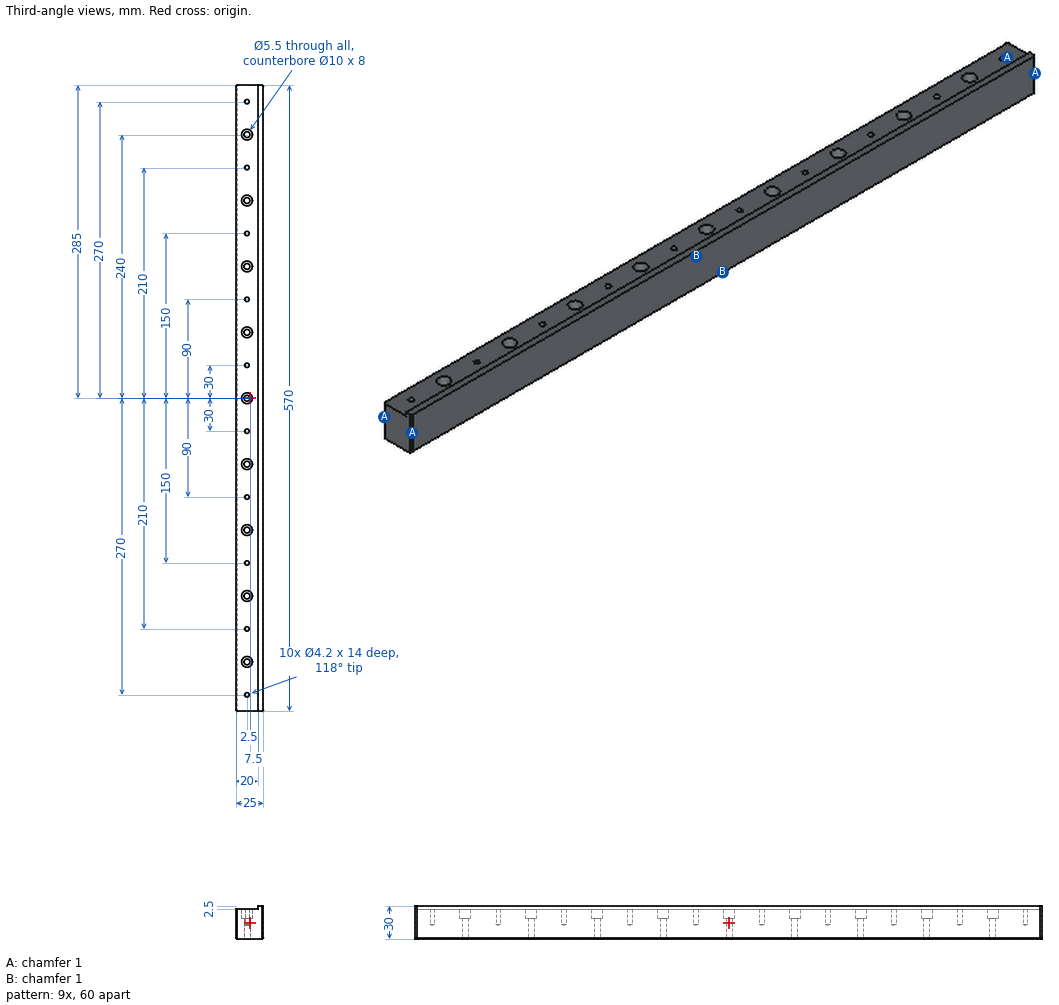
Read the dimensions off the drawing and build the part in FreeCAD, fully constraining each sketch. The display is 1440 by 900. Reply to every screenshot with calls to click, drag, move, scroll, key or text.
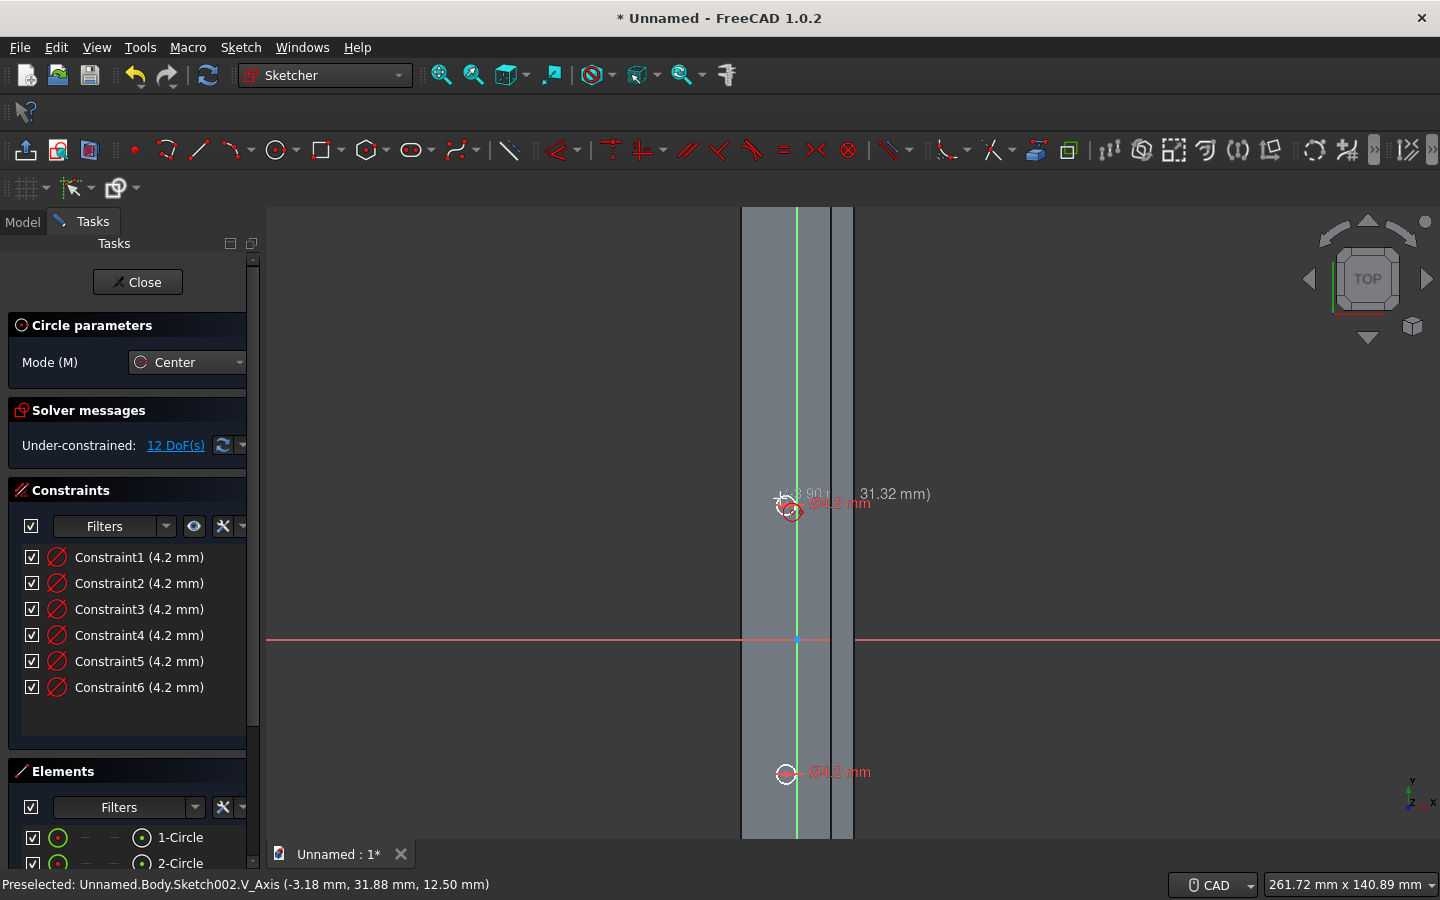
scroll(786, 236, up, 5)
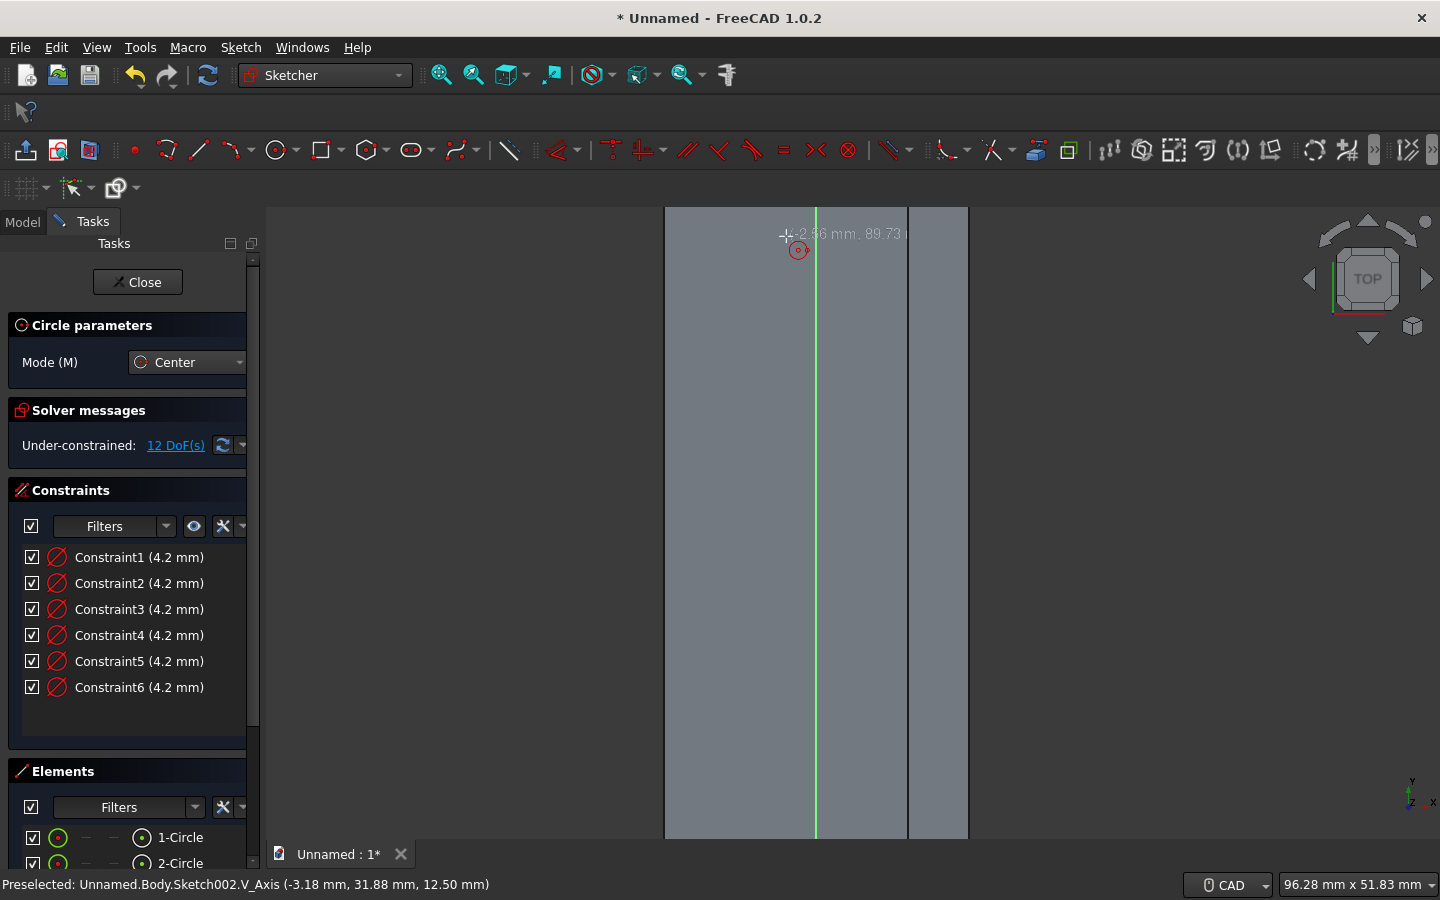
click(786, 235)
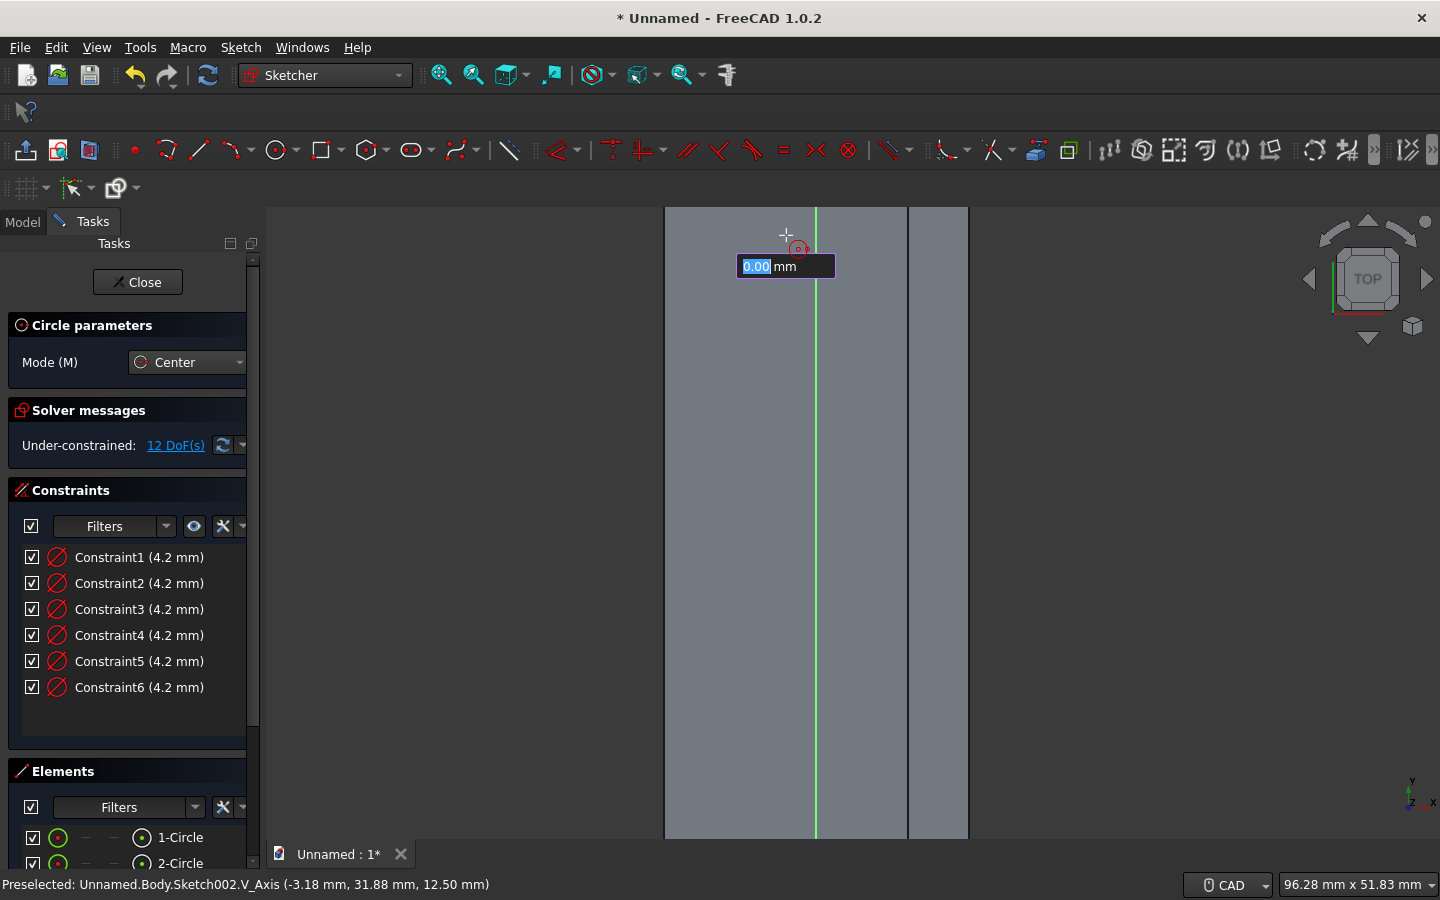
scroll(784, 471, down, 14)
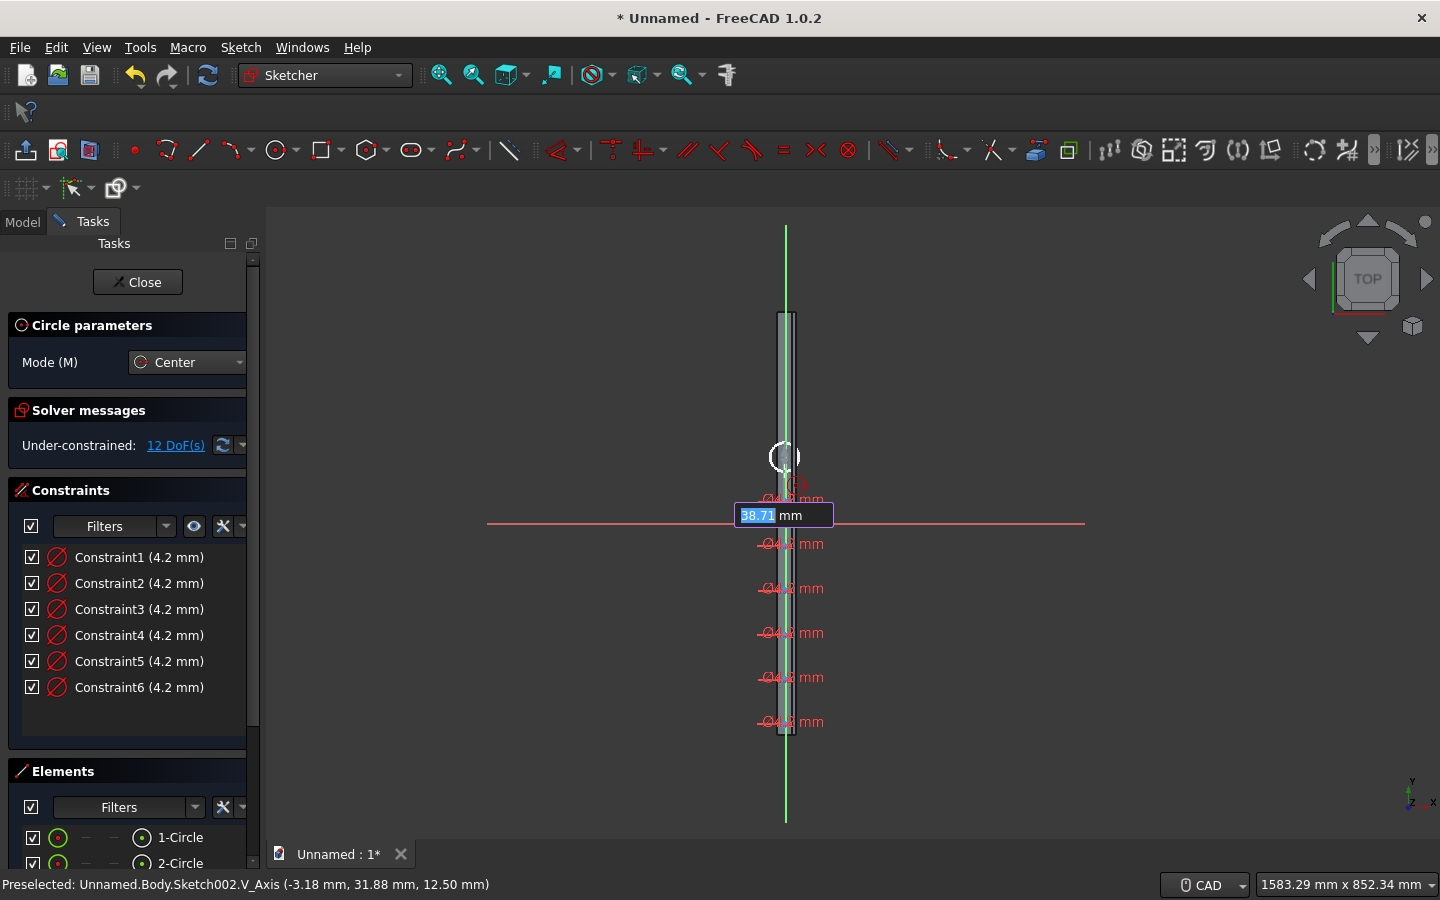
scroll(783, 456, up, 9)
move(783, 454)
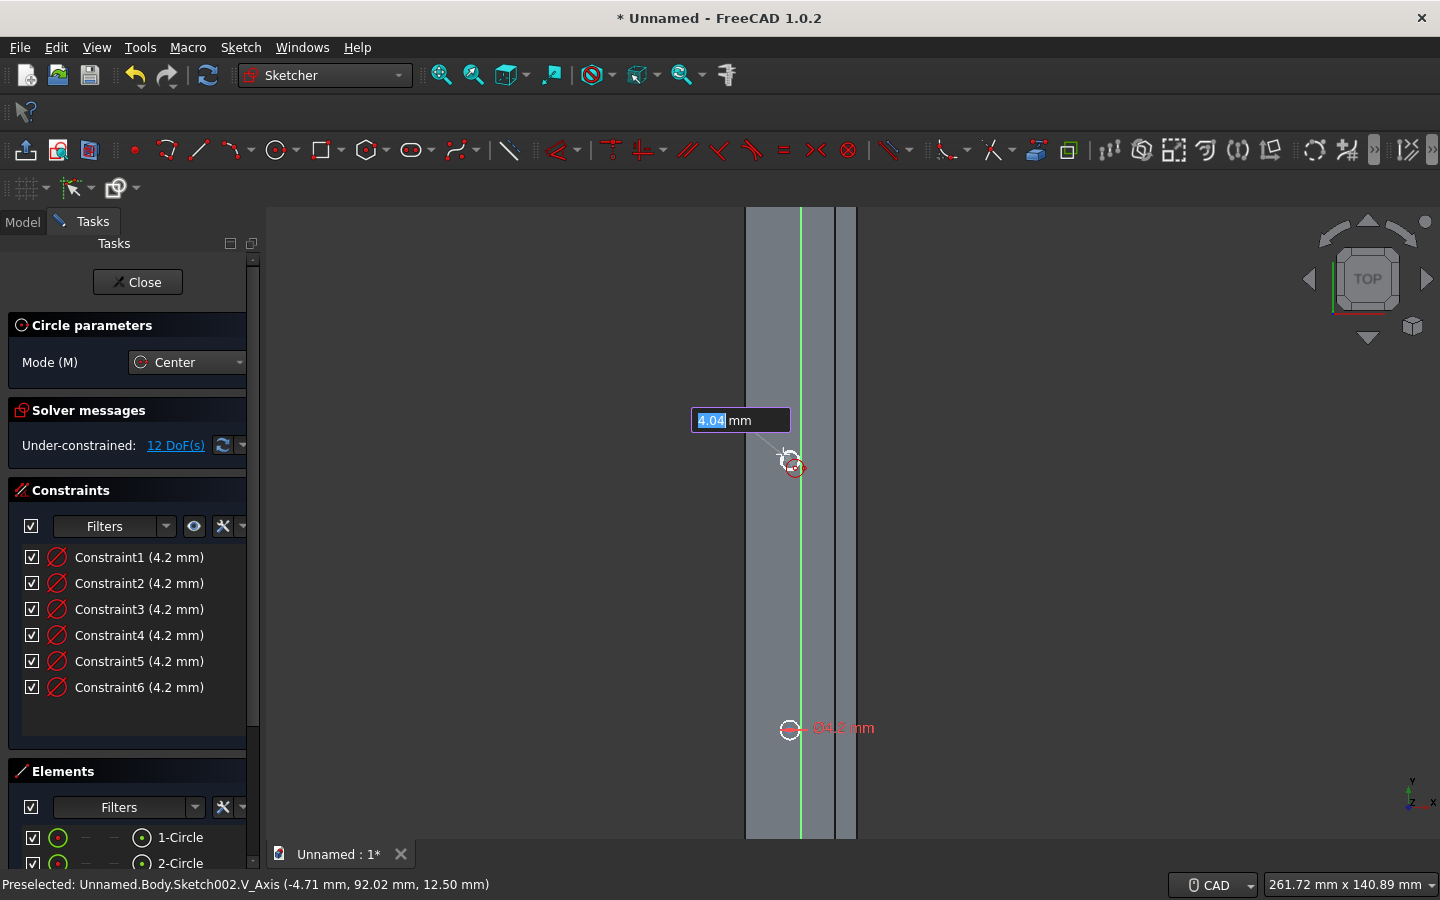
text(4.2)
key(Return)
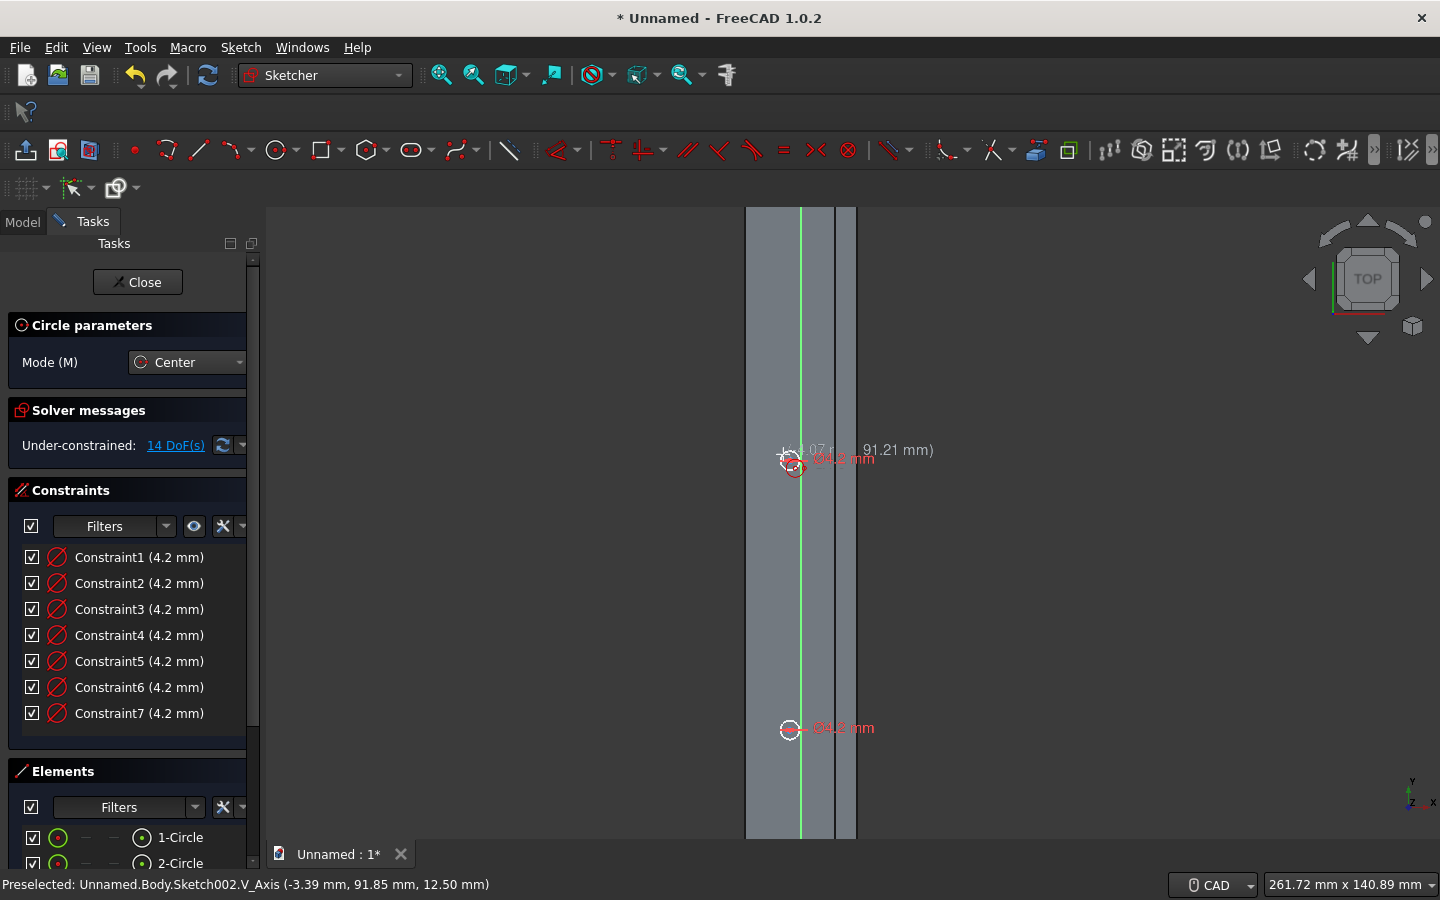
scroll(783, 455, down, 9)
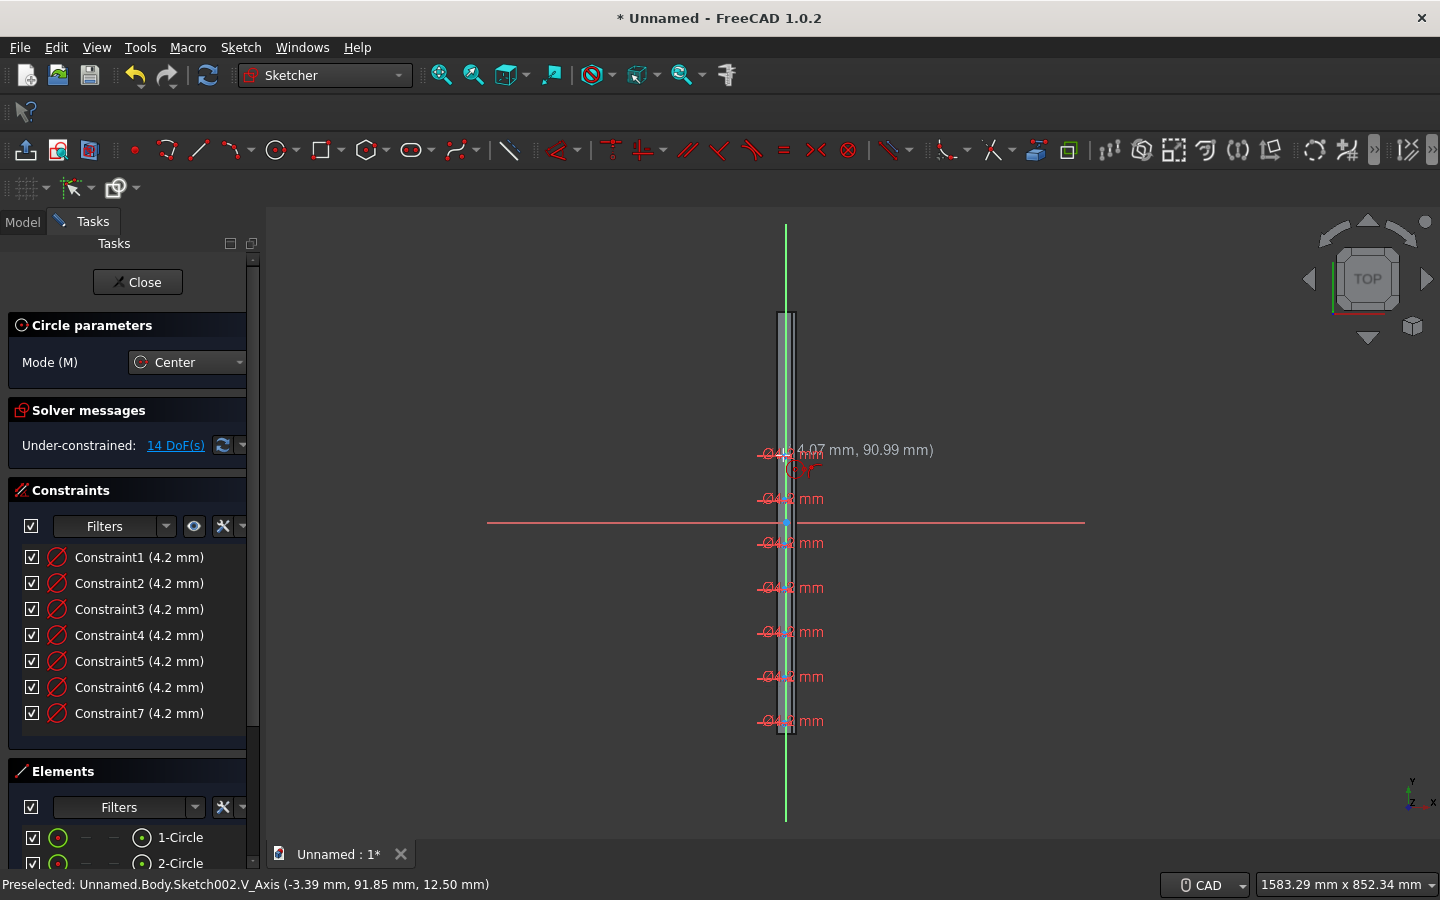
scroll(785, 412, up, 14)